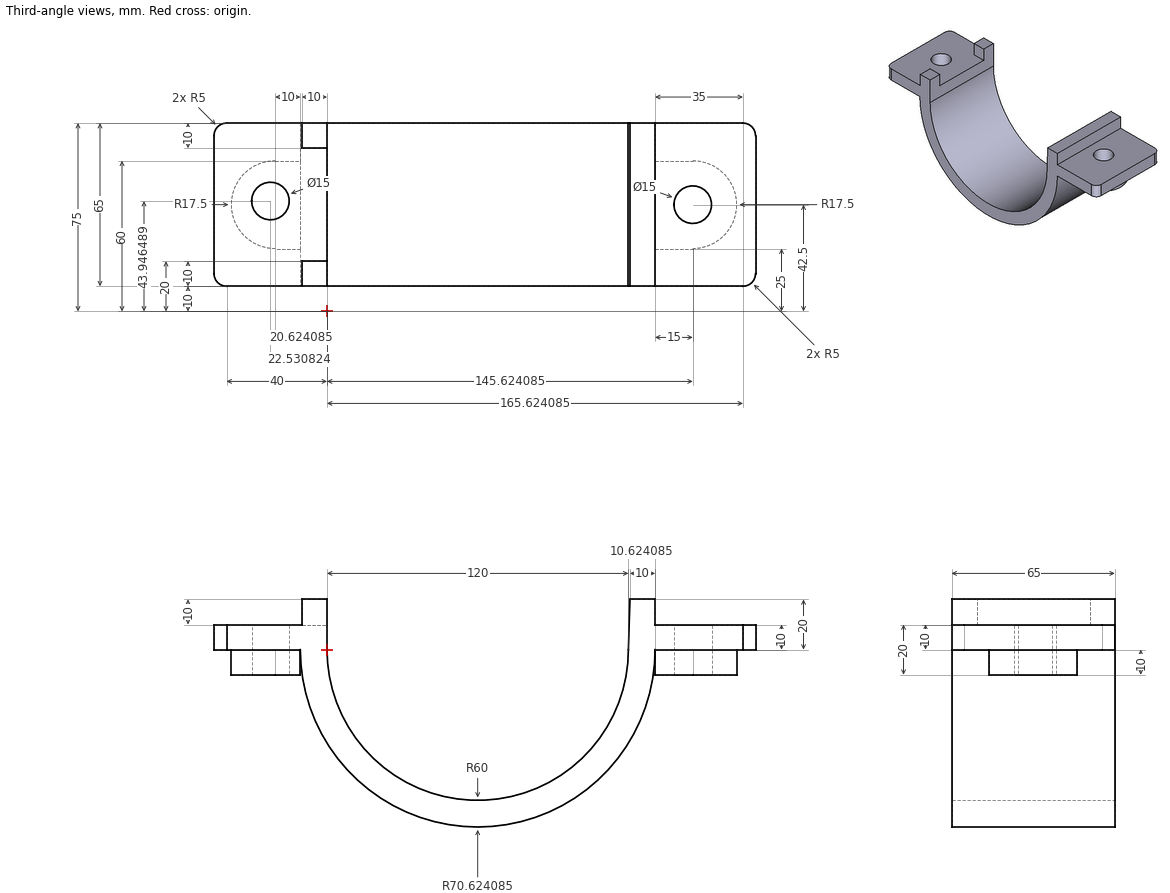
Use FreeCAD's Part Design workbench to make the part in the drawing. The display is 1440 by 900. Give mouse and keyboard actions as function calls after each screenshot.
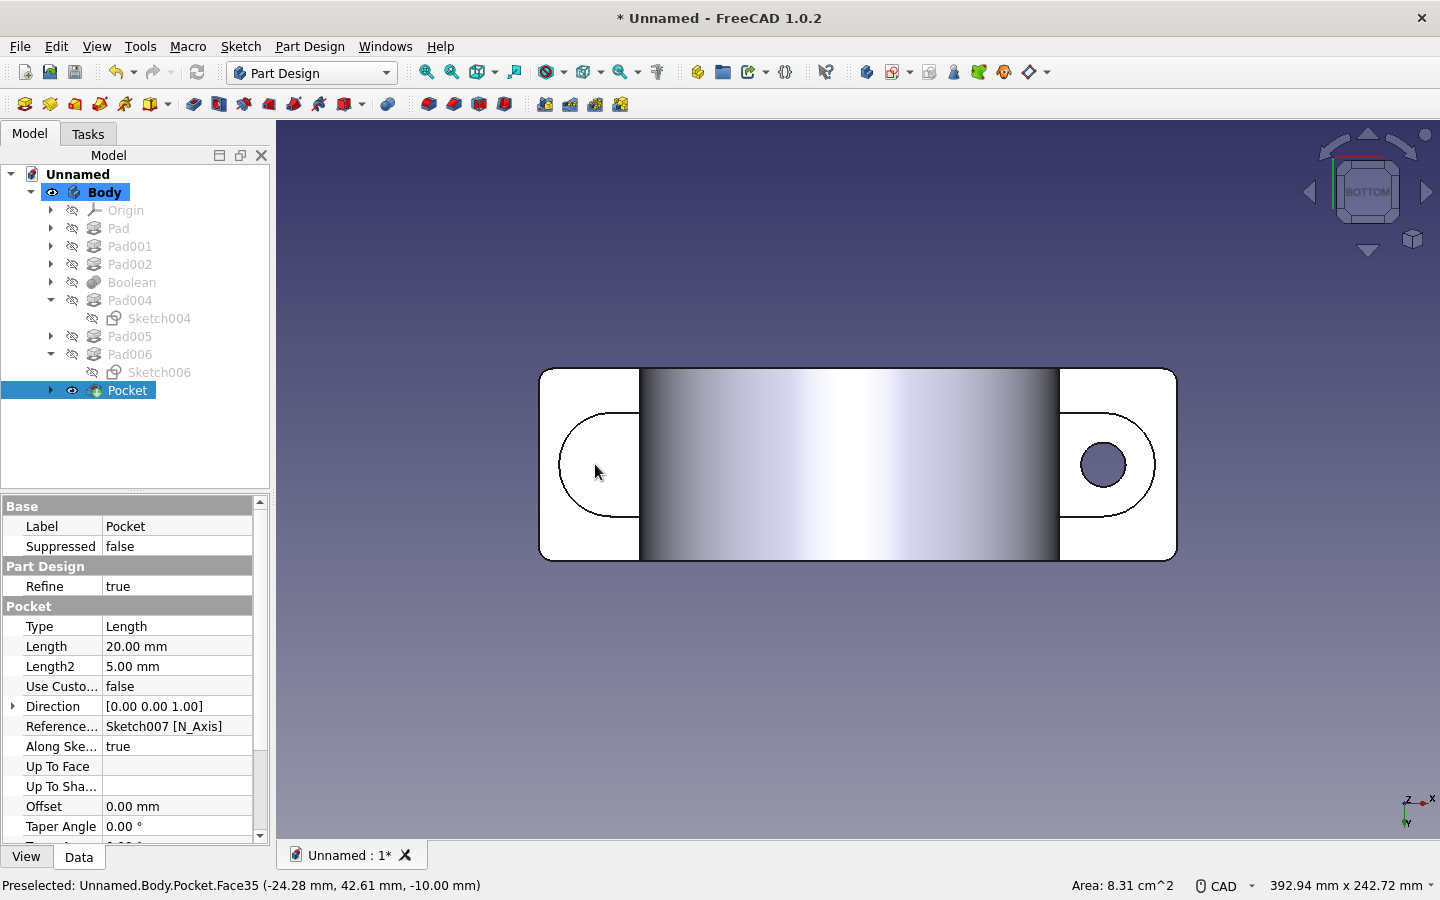
click(892, 72)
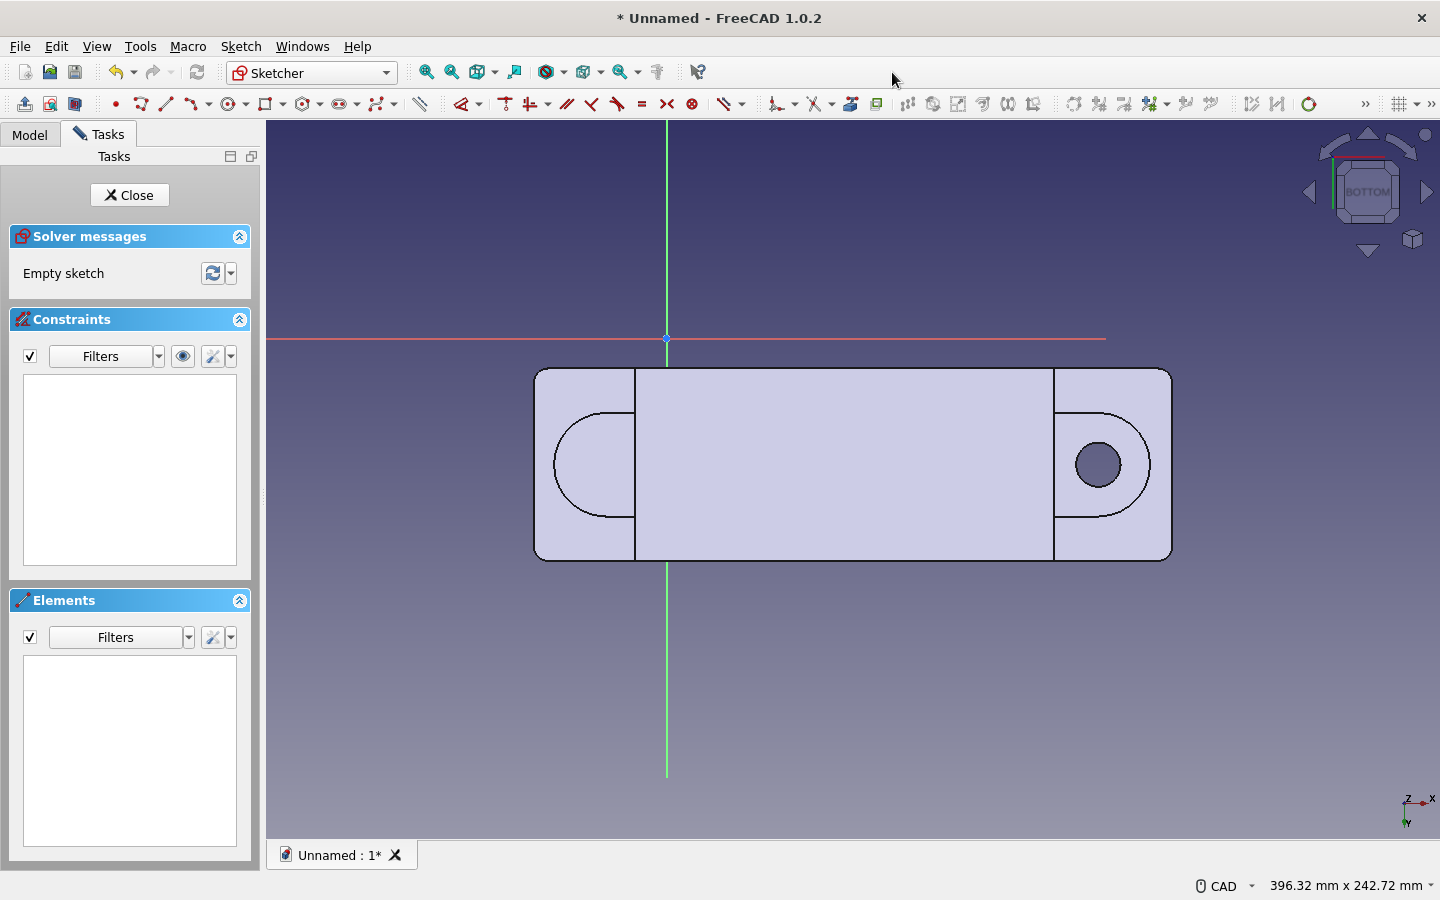
key(q)
key(s)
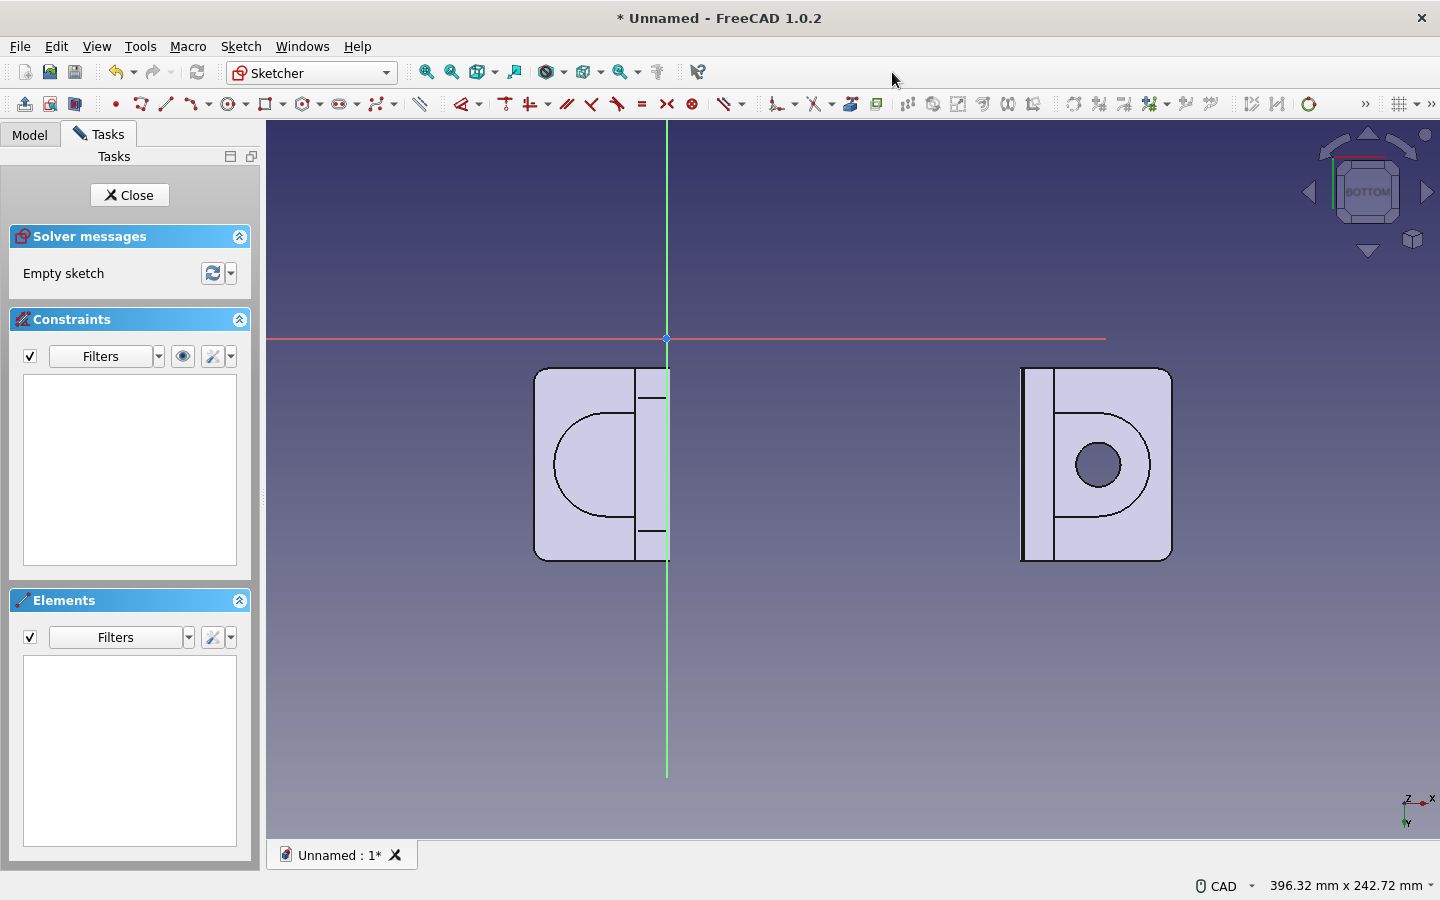
scroll(582, 468, up, 12)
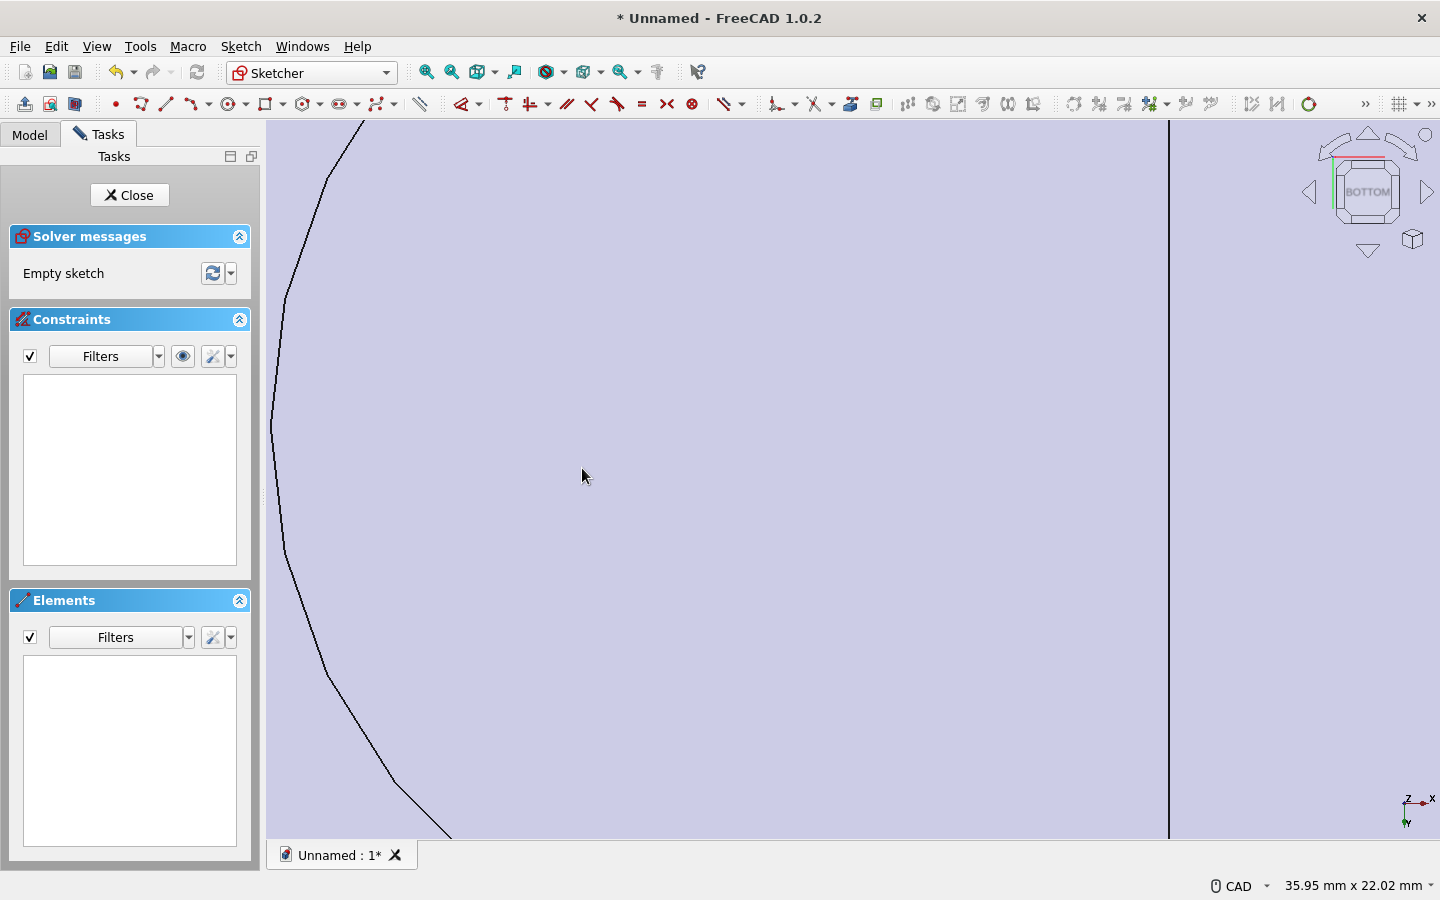
click(228, 104)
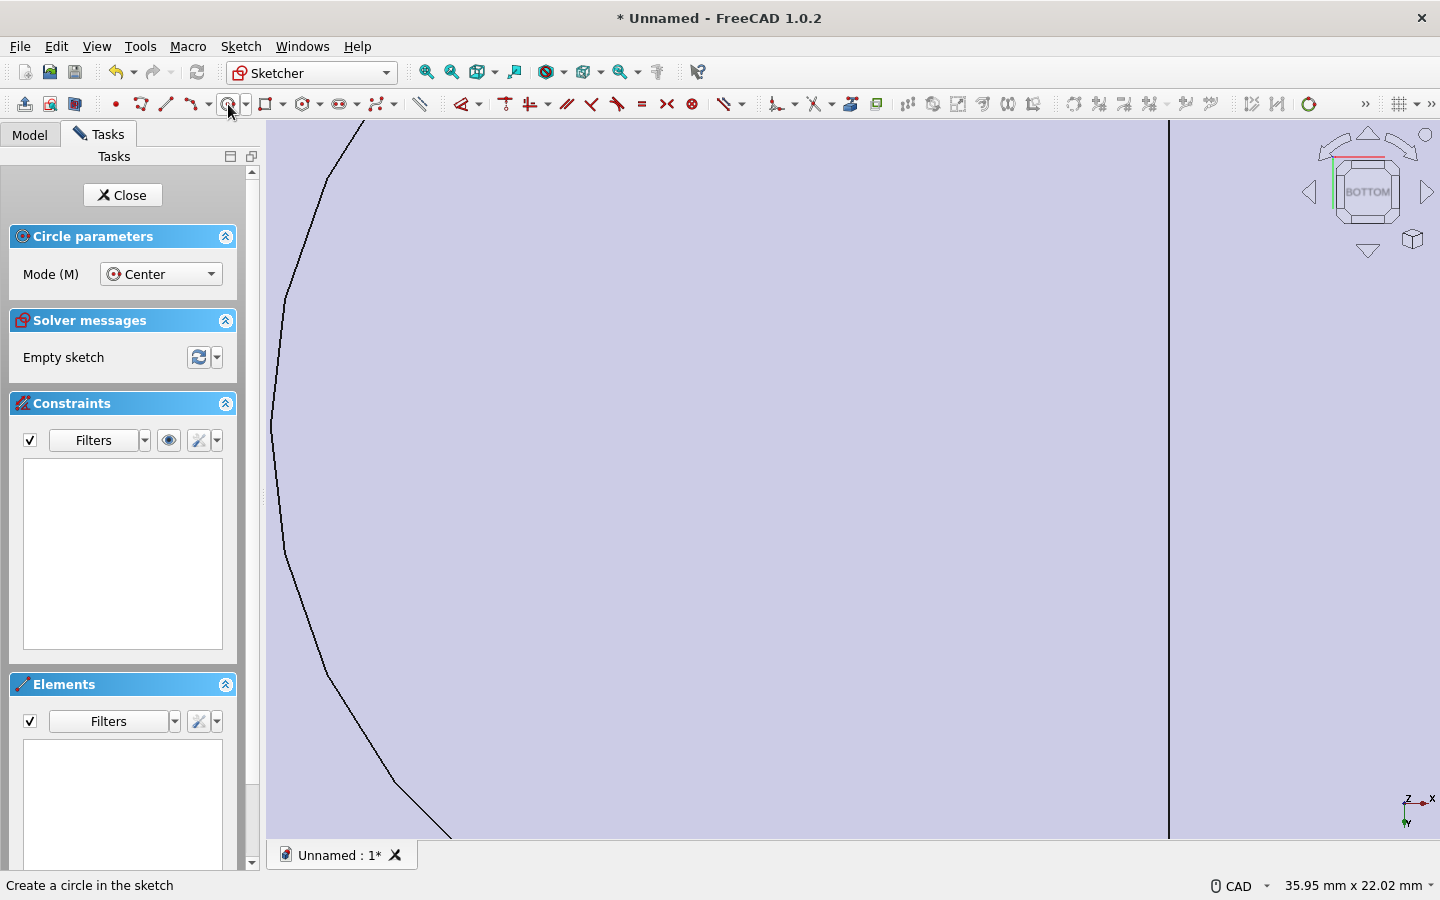
click(780, 474)
move(953, 301)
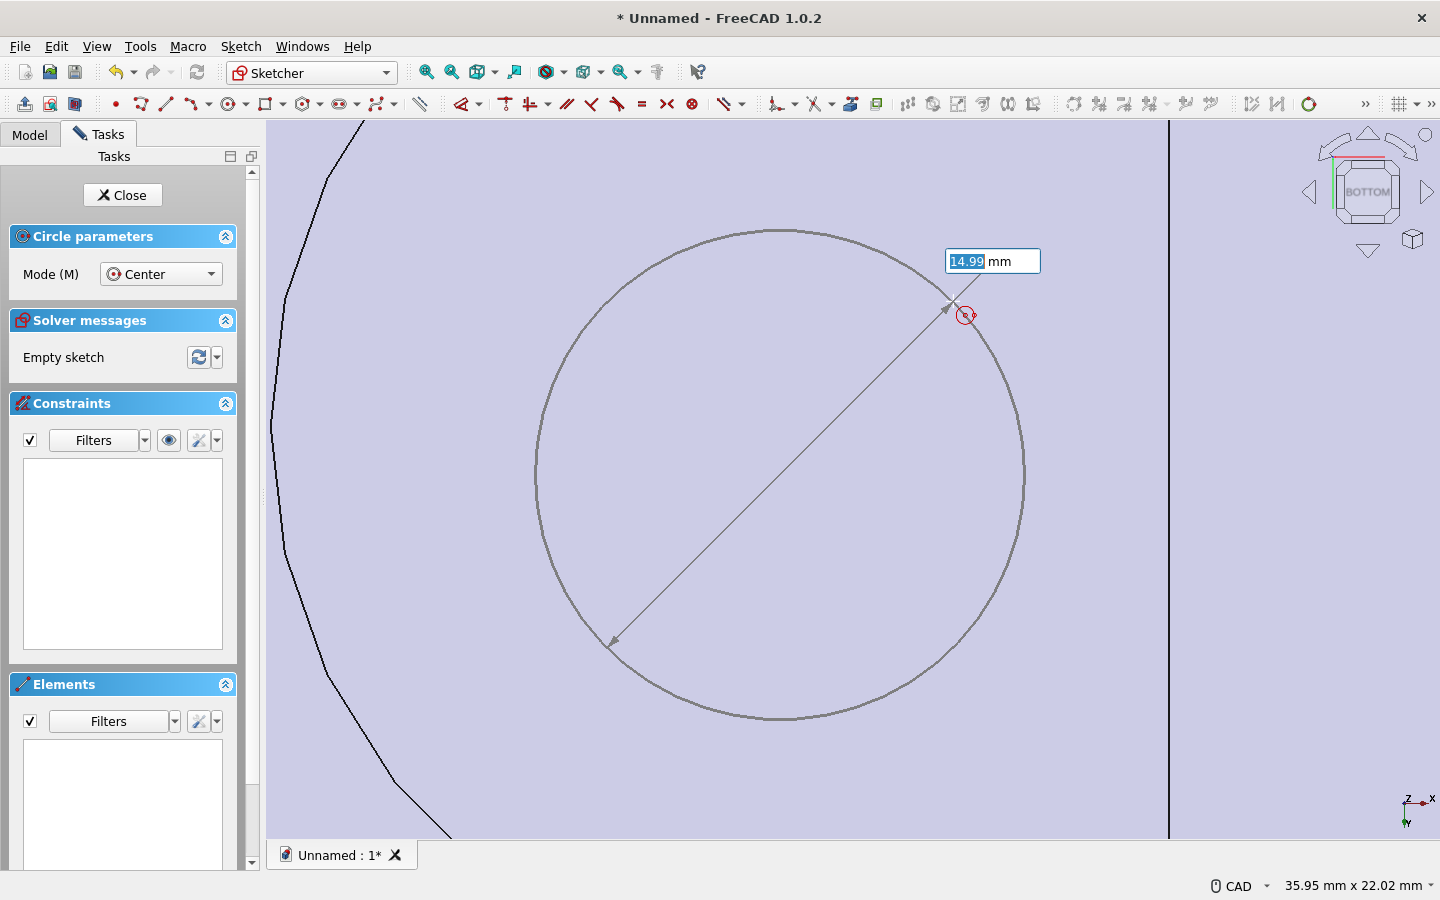
text(15)
key(Return)
key(Escape)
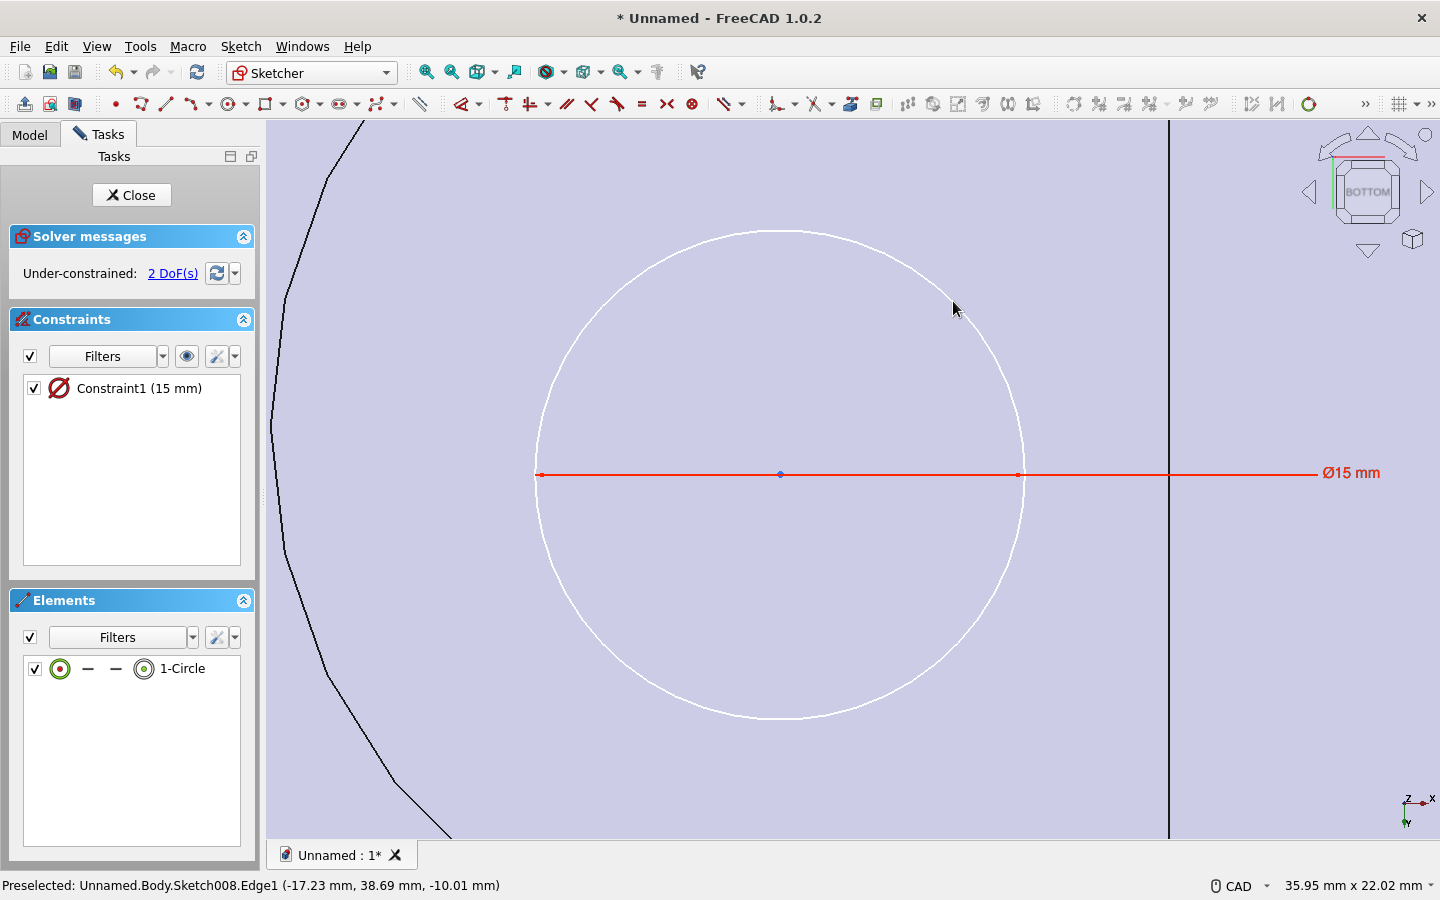
click(460, 104)